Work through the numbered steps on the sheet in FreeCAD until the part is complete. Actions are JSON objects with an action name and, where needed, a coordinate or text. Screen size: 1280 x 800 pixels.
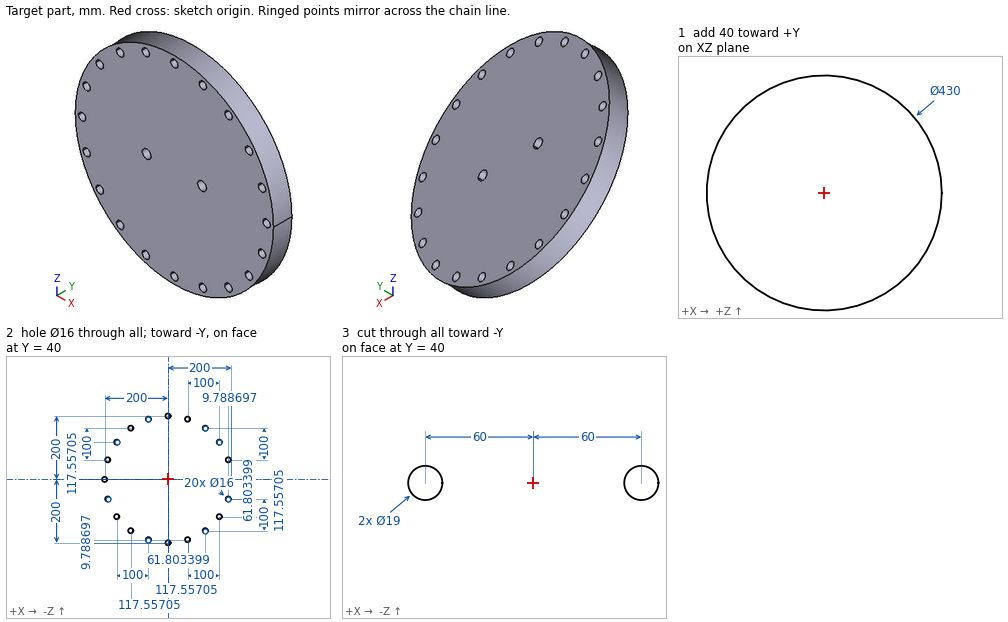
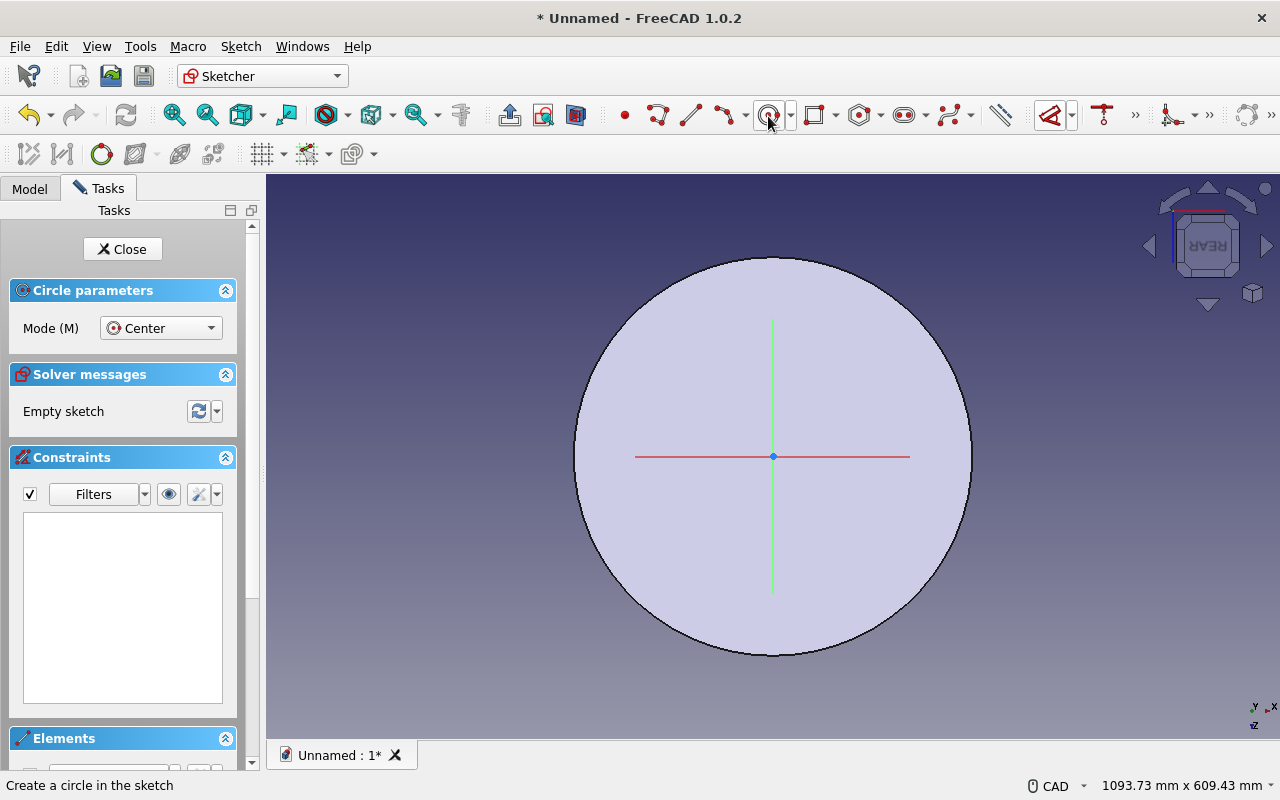
{"action": "scroll", "coordinate": [958, 456], "scroll_direction": "up", "scroll_amount": 6}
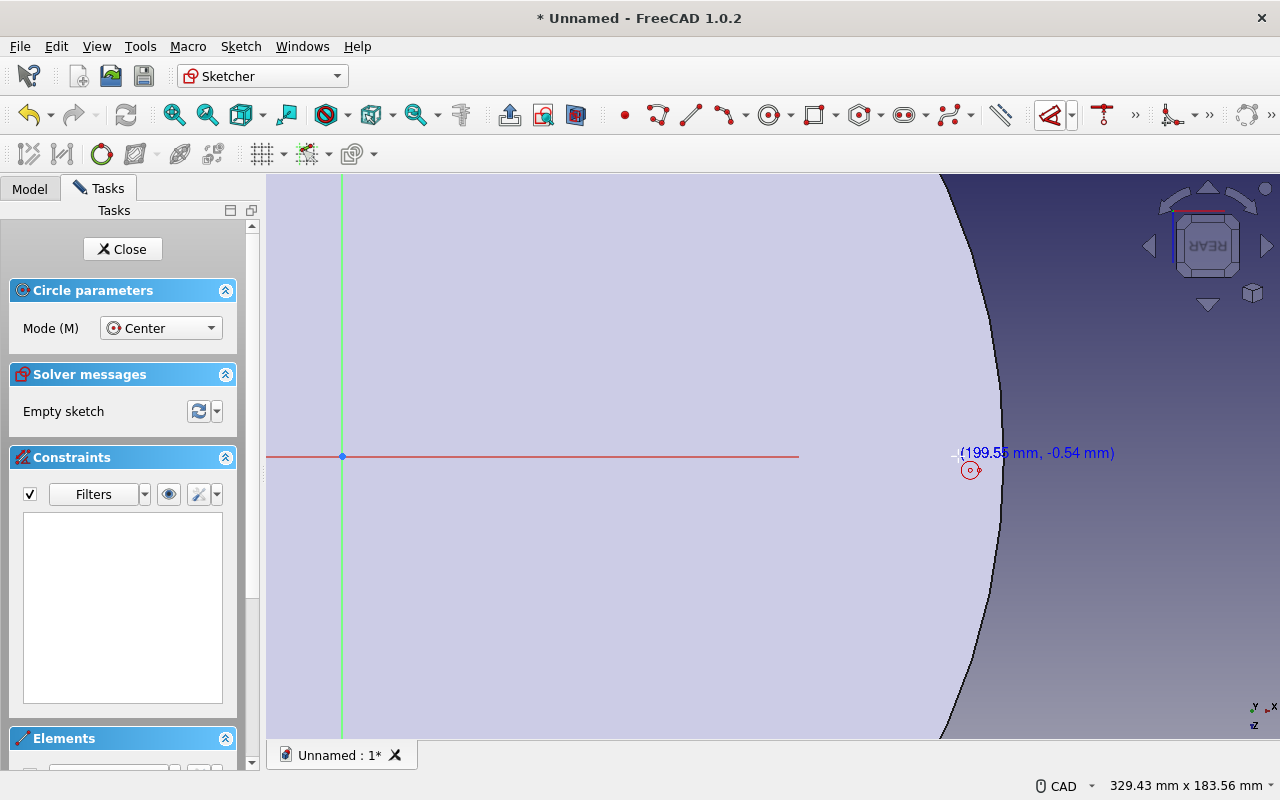
{"action": "left_click", "coordinate": [958, 456]}
{"action": "left_click", "coordinate": [975, 439]}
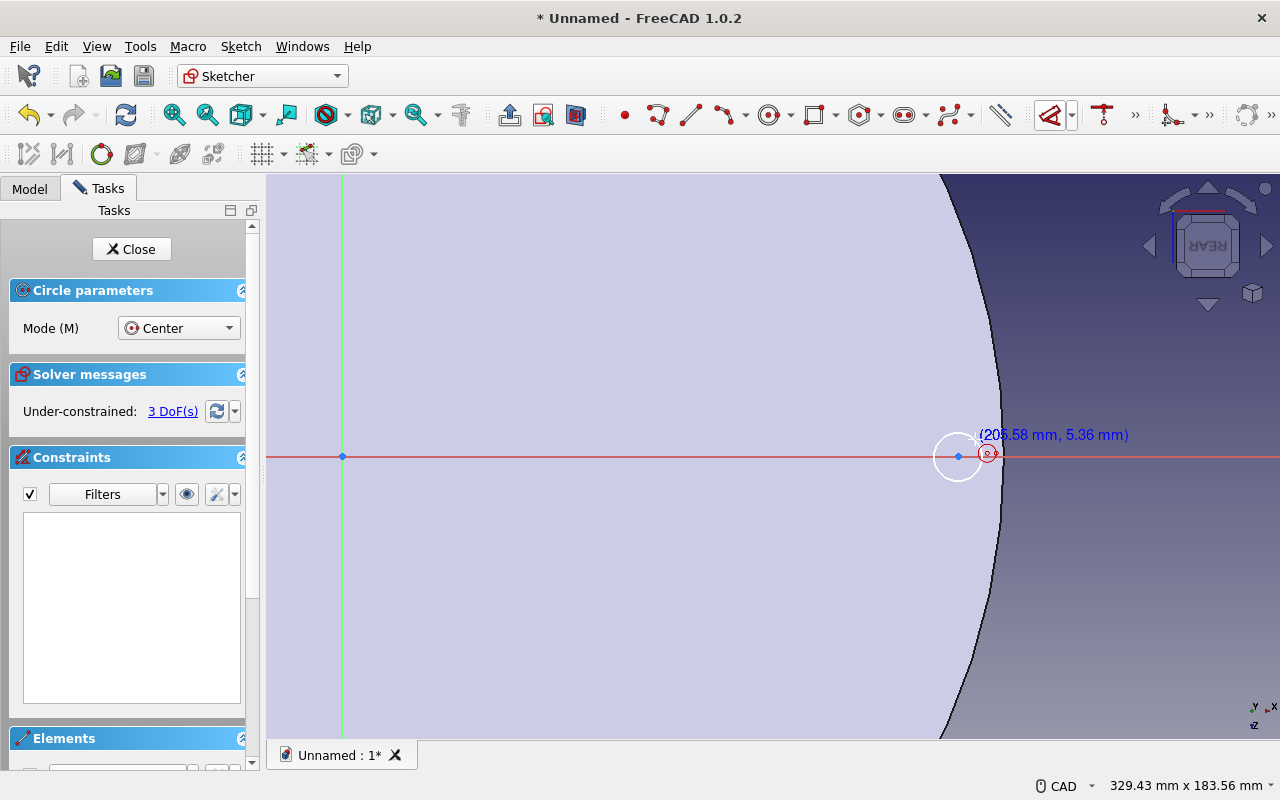
{"action": "left_click", "coordinate": [928, 647]}
{"action": "left_click", "coordinate": [945, 629]}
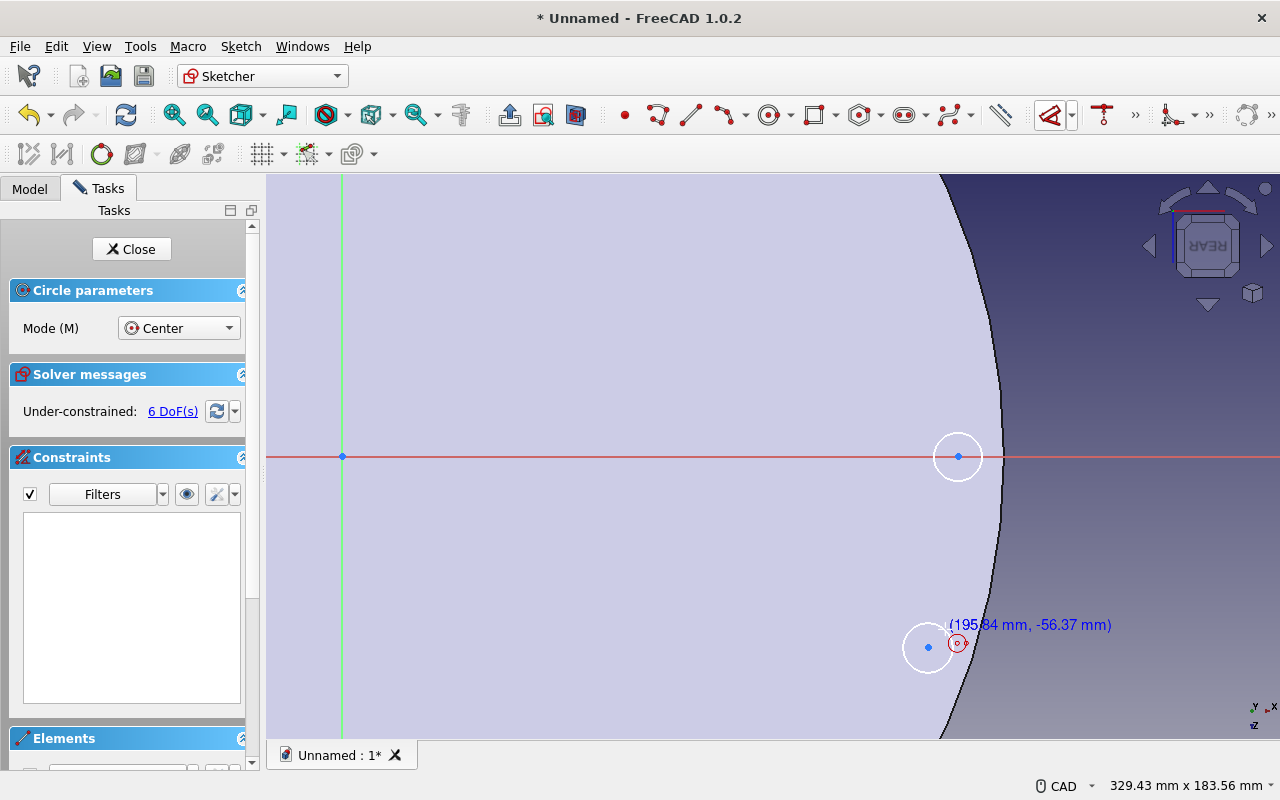
{"action": "scroll", "coordinate": [861, 457], "scroll_direction": "down", "scroll_amount": 6}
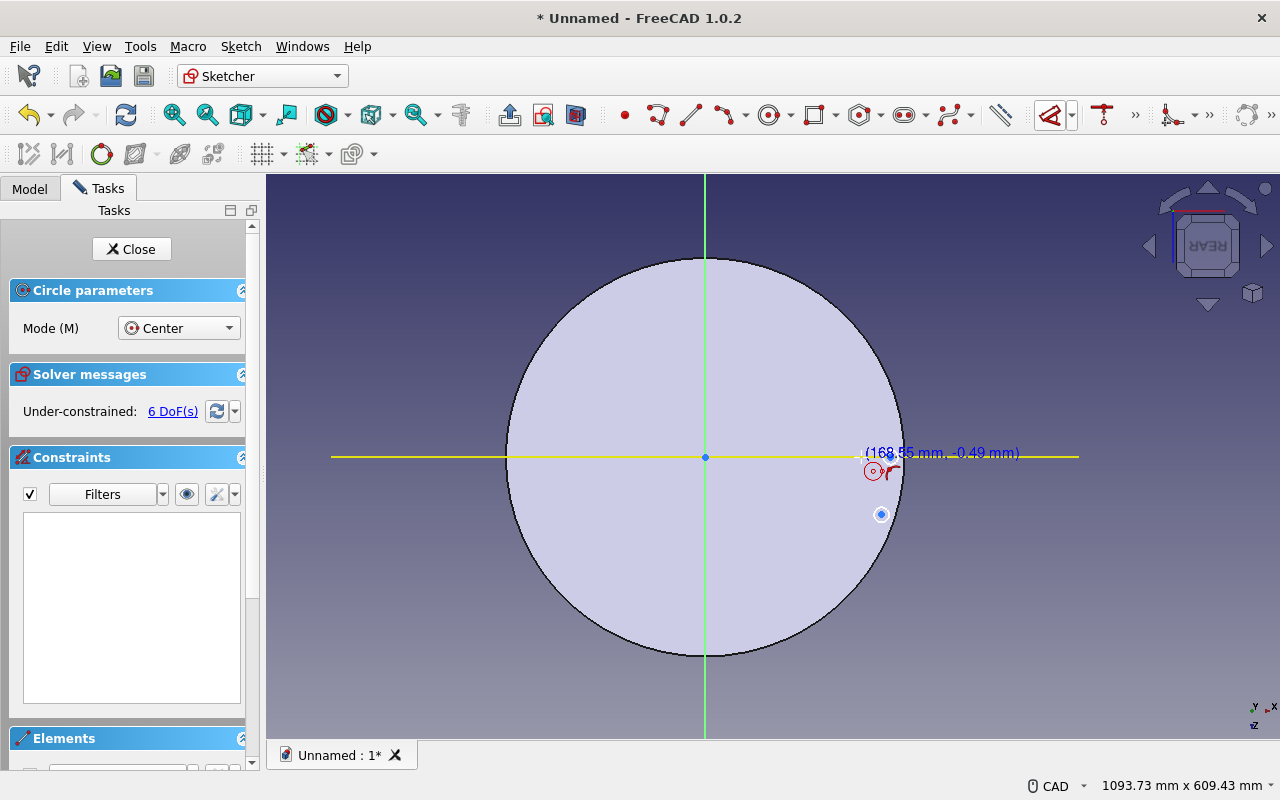
{"action": "scroll", "coordinate": [855, 566], "scroll_direction": "up", "scroll_amount": 6}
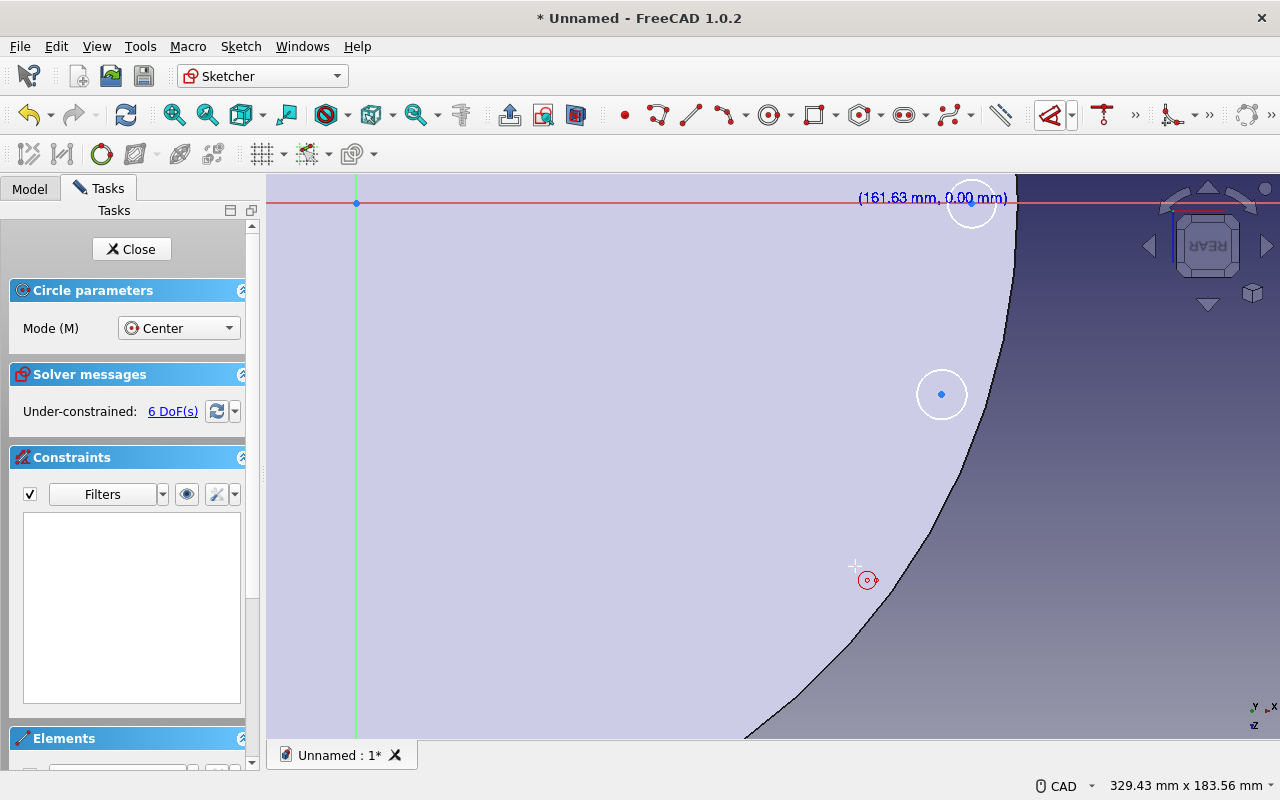
{"action": "left_click", "coordinate": [854, 565]}
{"action": "left_click", "coordinate": [872, 548]}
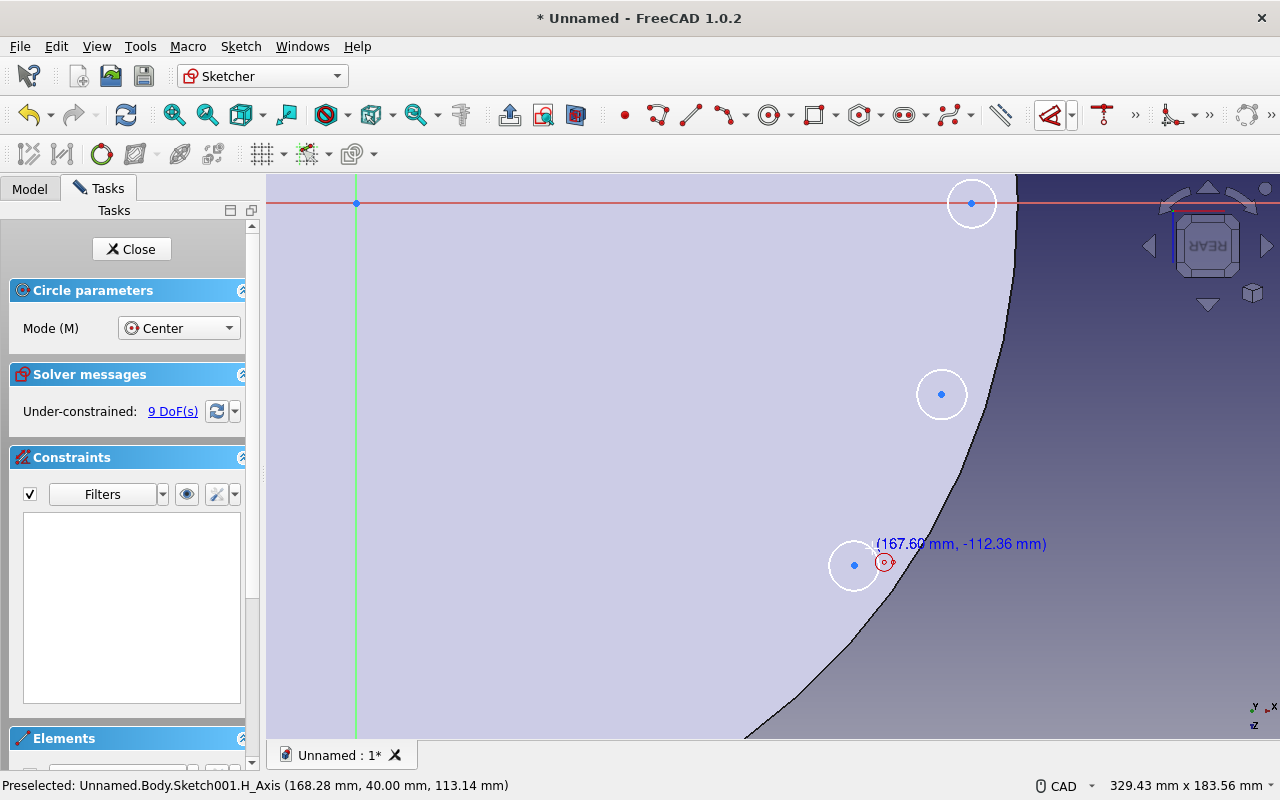
{"action": "left_click", "coordinate": [718, 701]}
{"action": "left_click", "coordinate": [735, 684]}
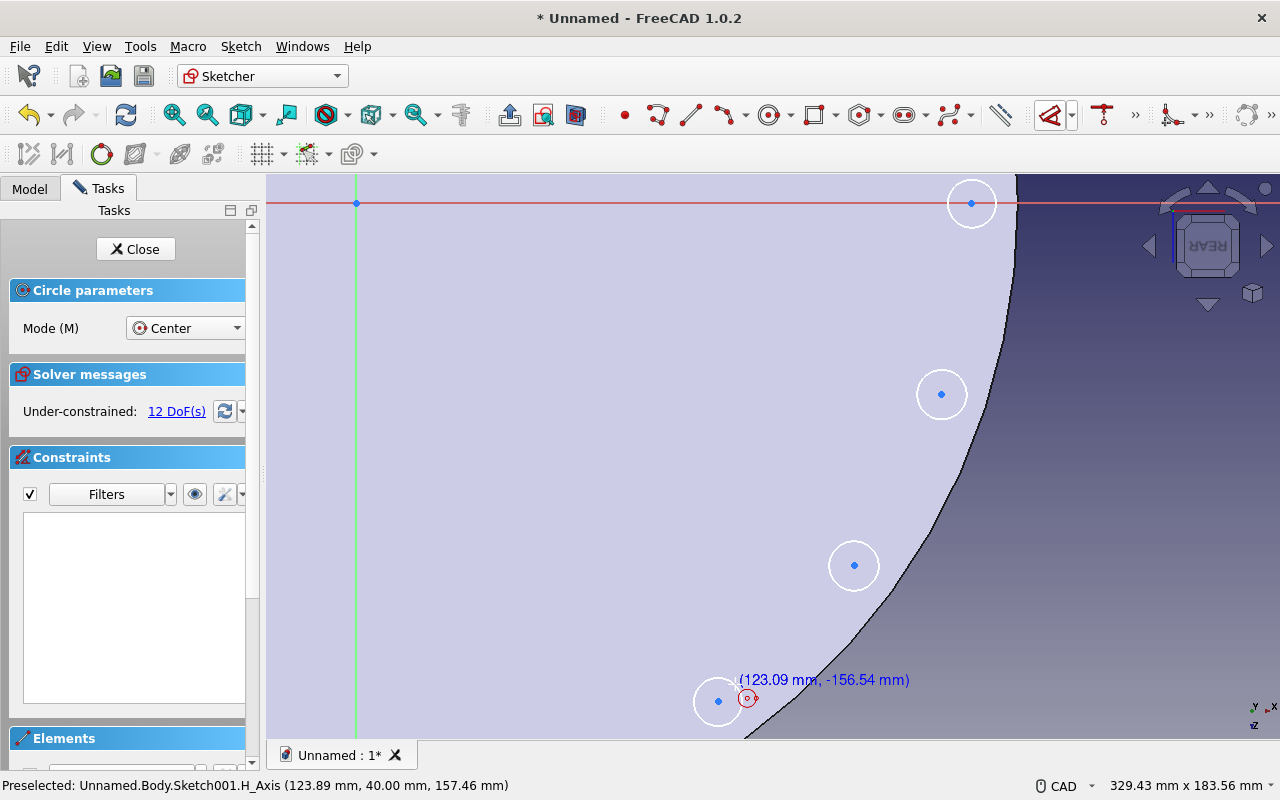
{"action": "scroll", "coordinate": [855, 566], "scroll_direction": "down", "scroll_amount": 6}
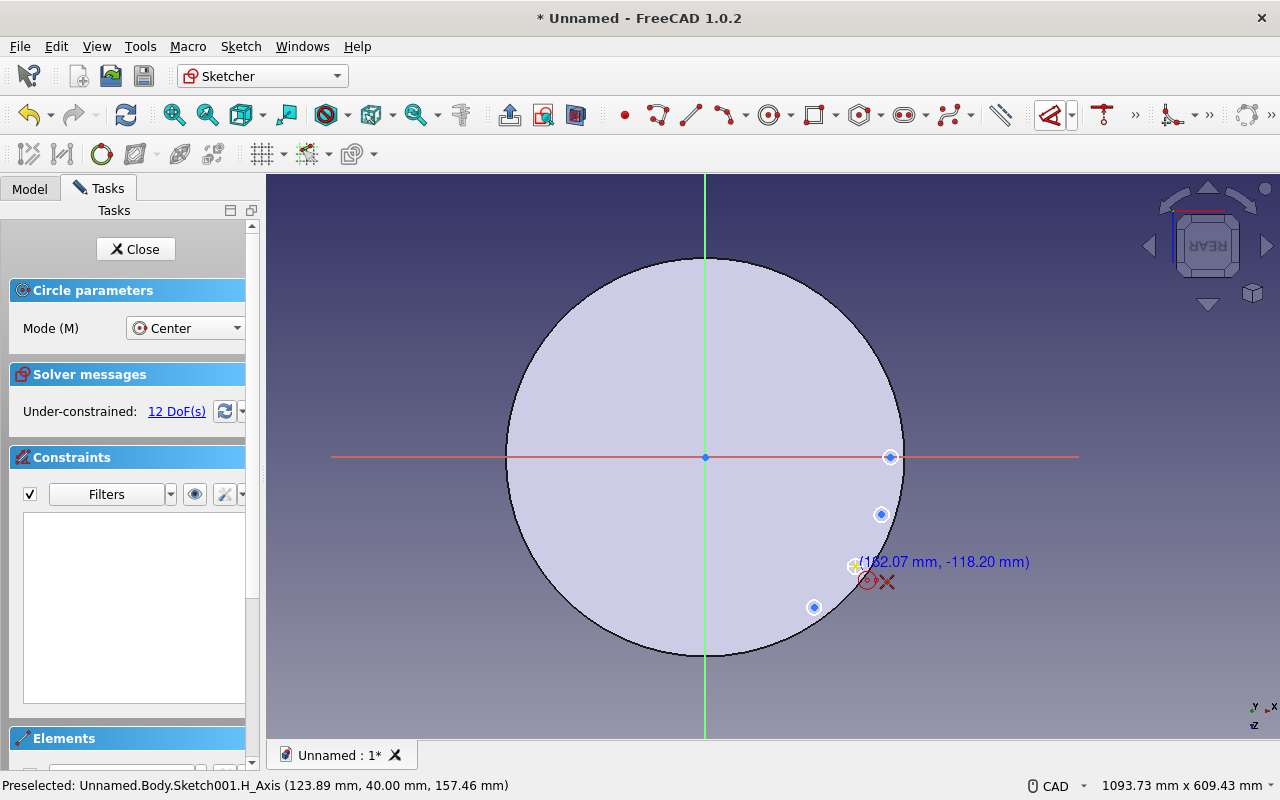
{"action": "scroll", "coordinate": [762, 634], "scroll_direction": "up", "scroll_amount": 6}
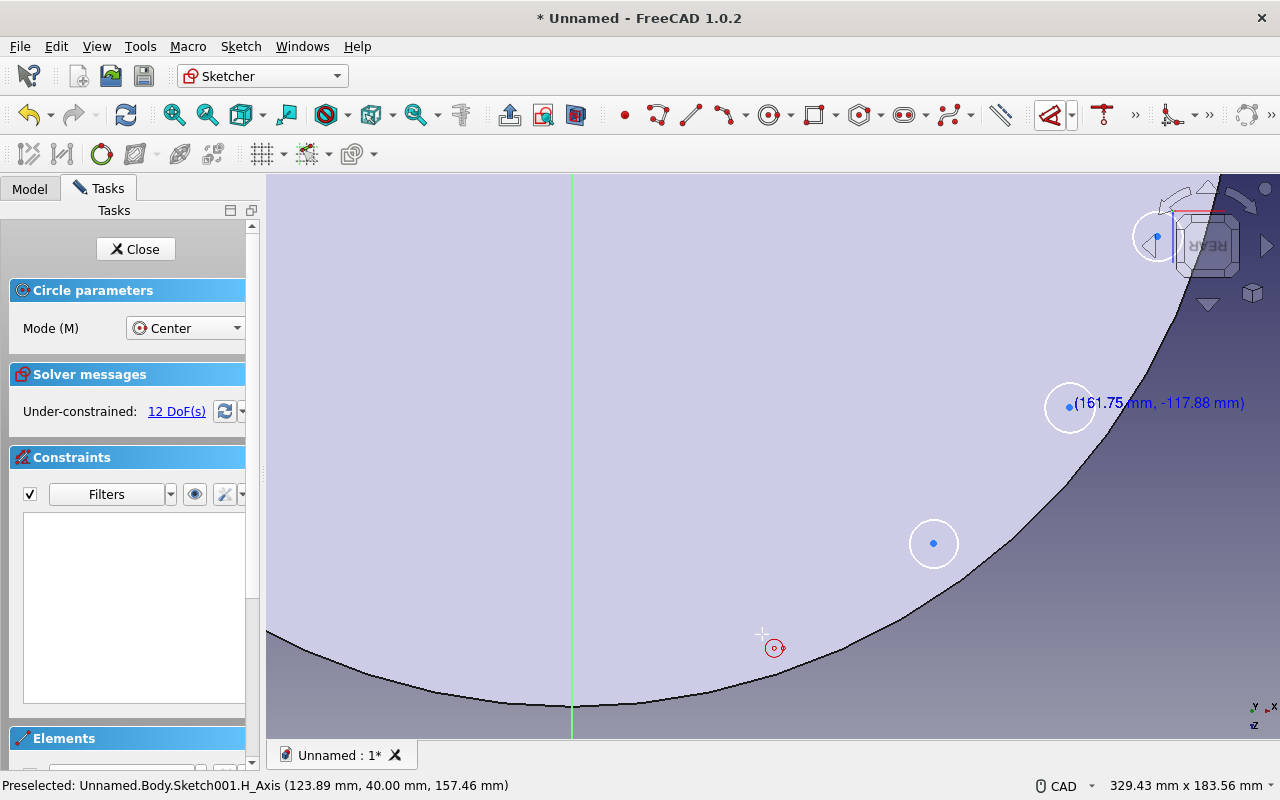
{"action": "left_click", "coordinate": [762, 631]}
{"action": "left_click", "coordinate": [780, 613]}